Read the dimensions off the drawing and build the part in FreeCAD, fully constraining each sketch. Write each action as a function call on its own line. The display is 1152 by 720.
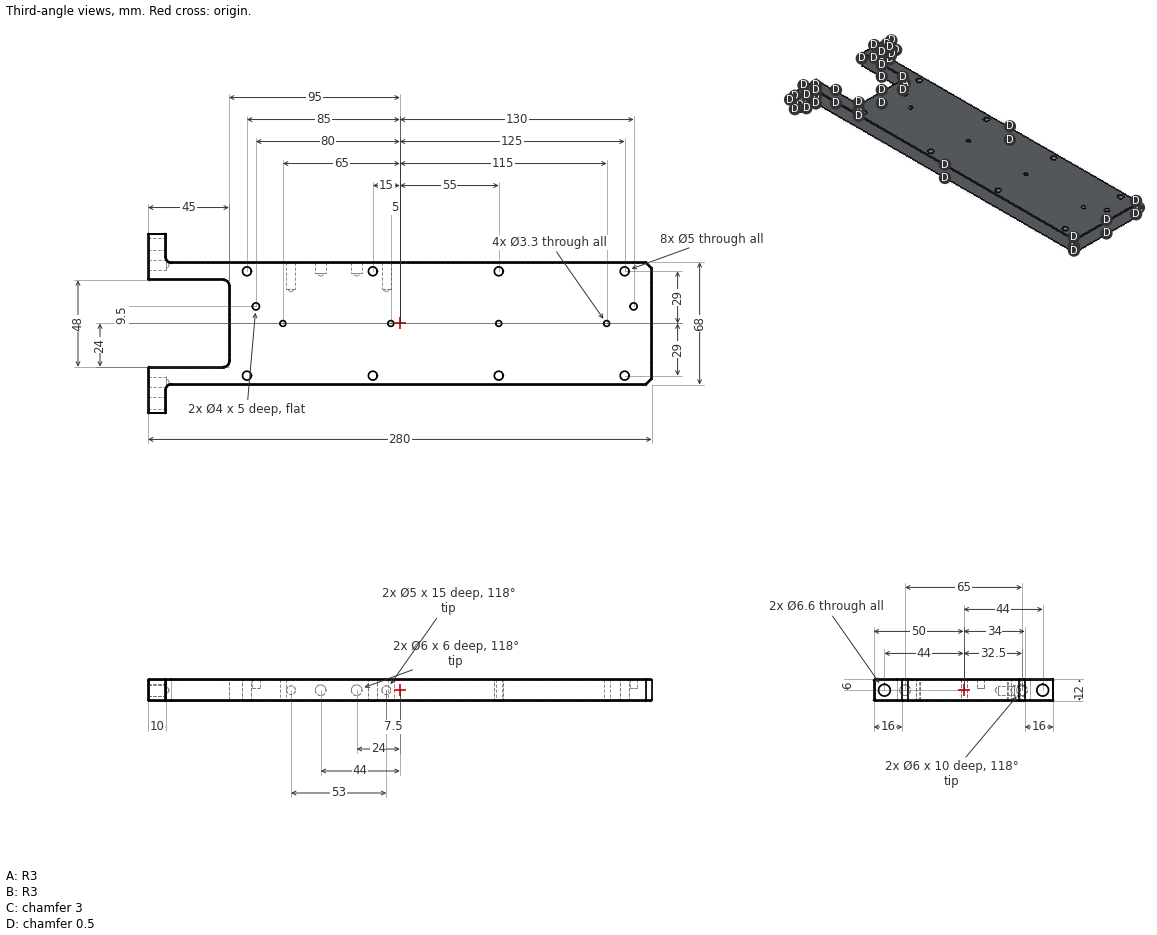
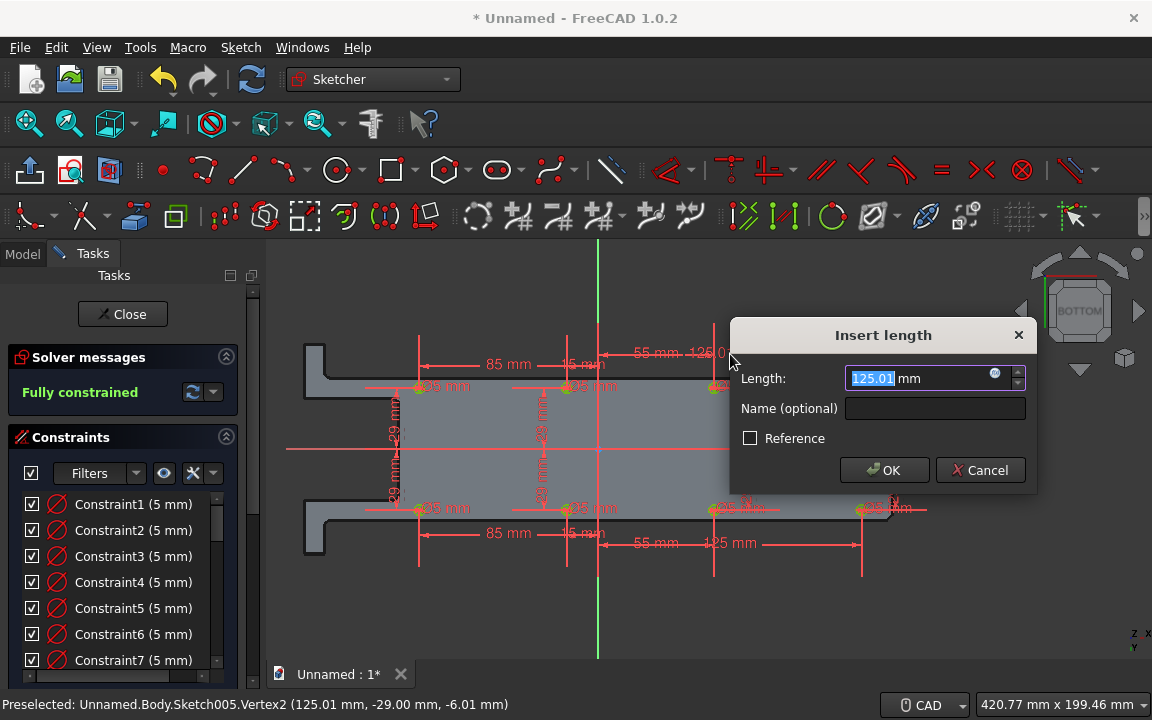
text(125)
key(Return)
key(Escape)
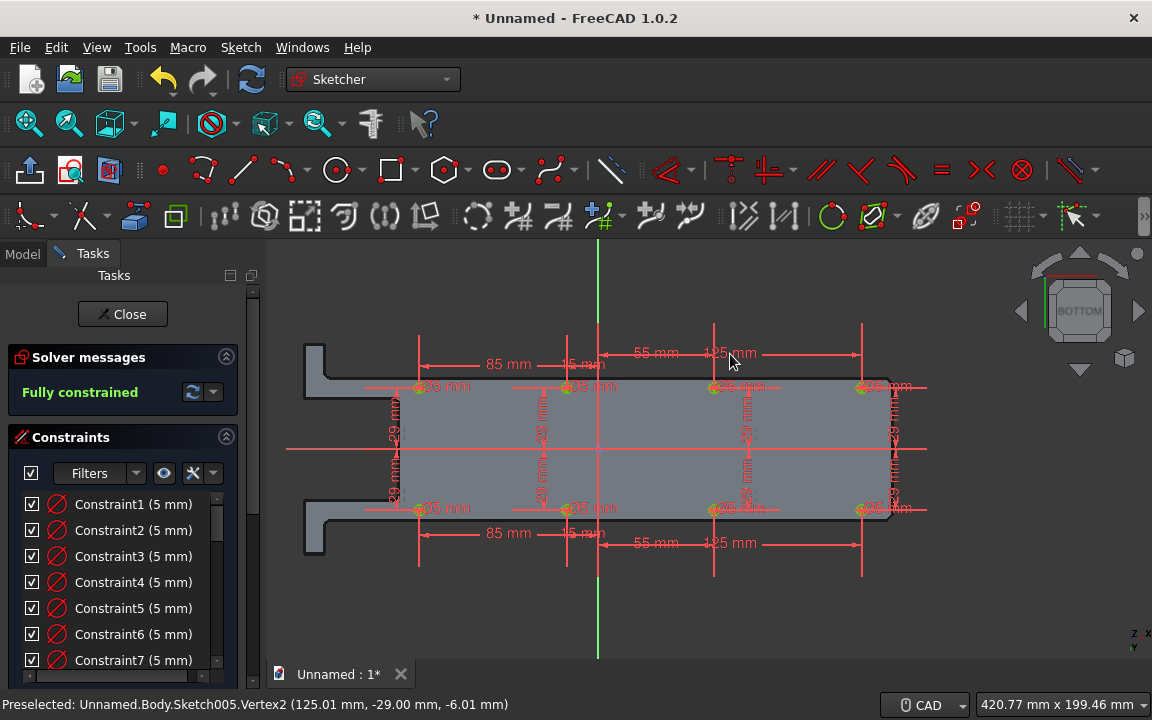
click(123, 314)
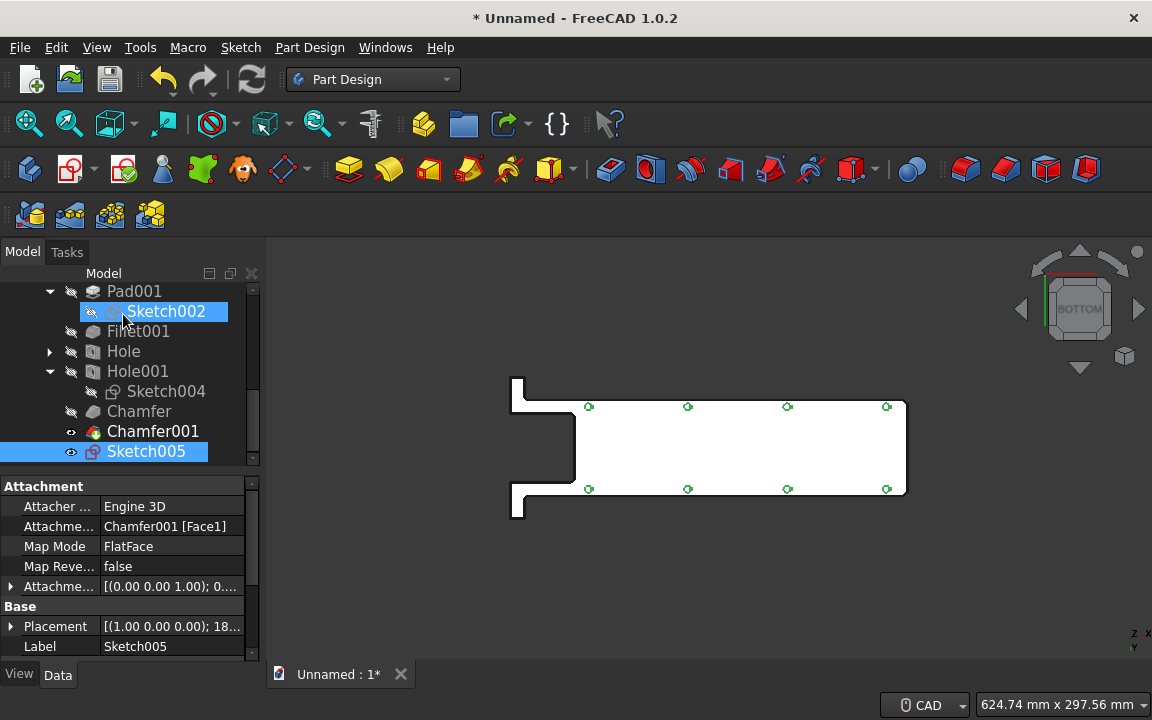
click(652, 170)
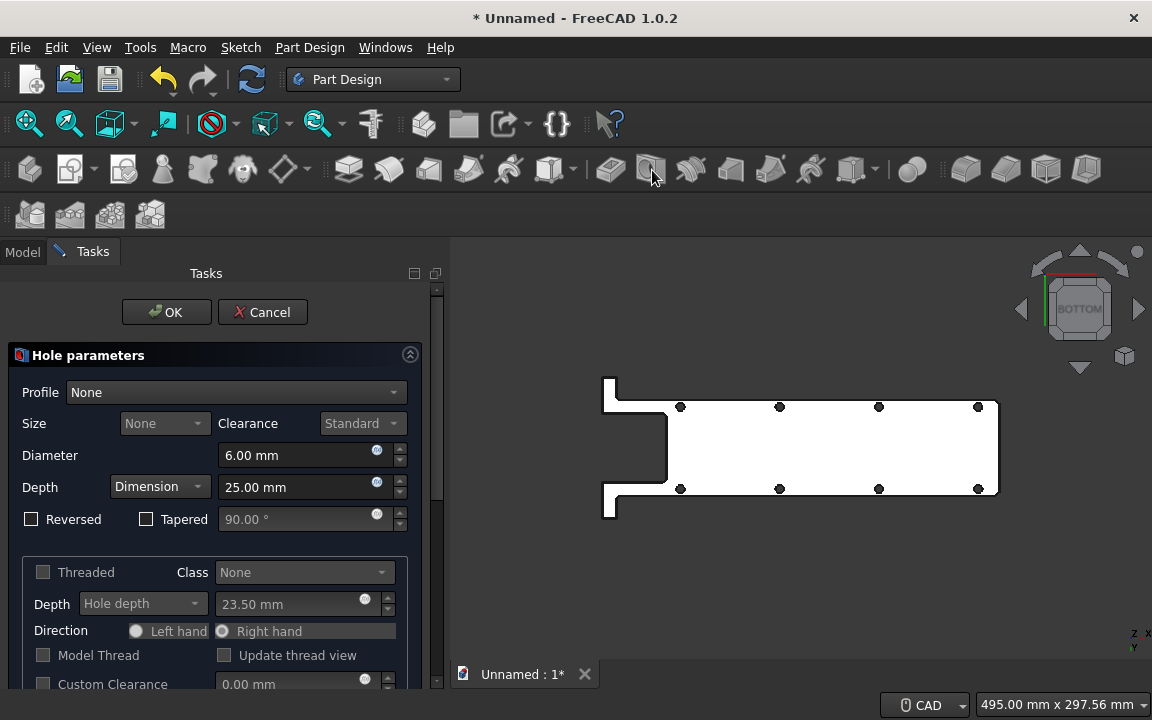
triple_click(305, 455)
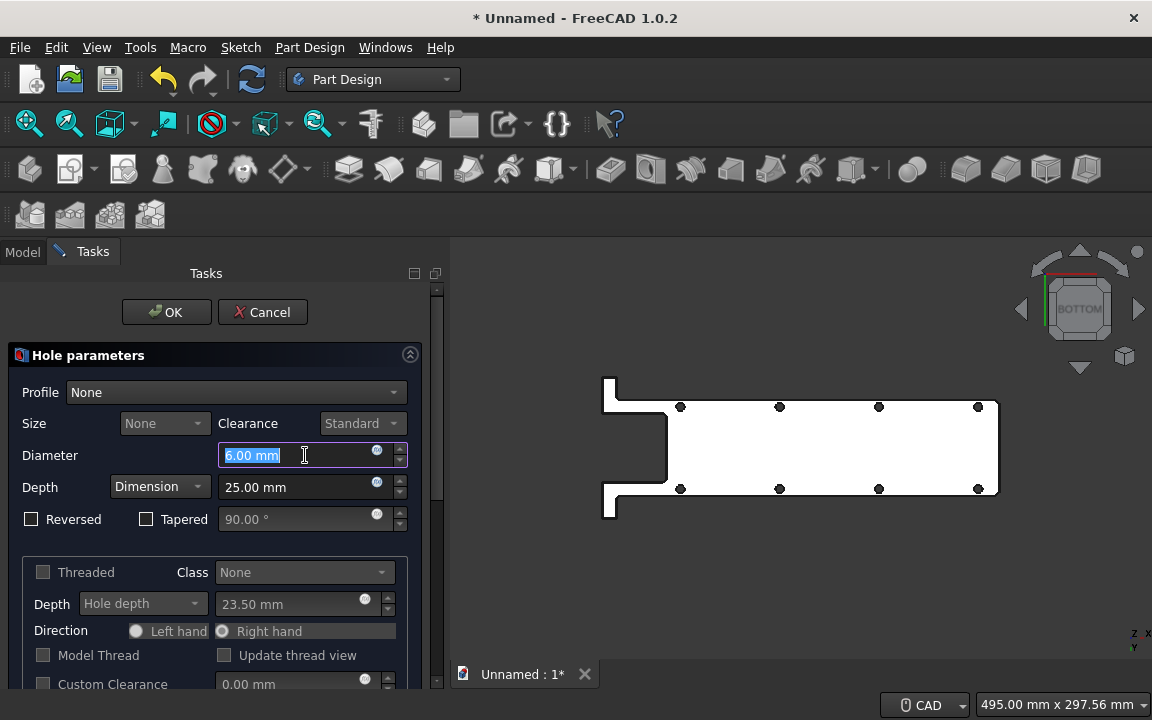
text(5)
key(Tab)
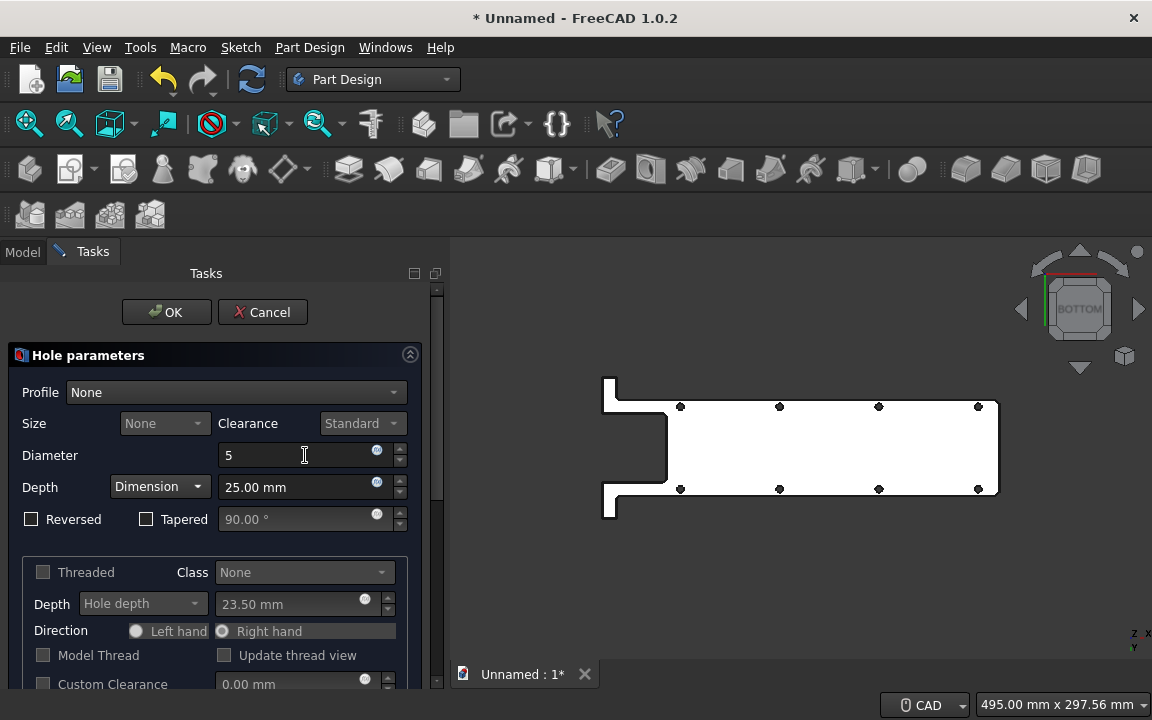
click(161, 486)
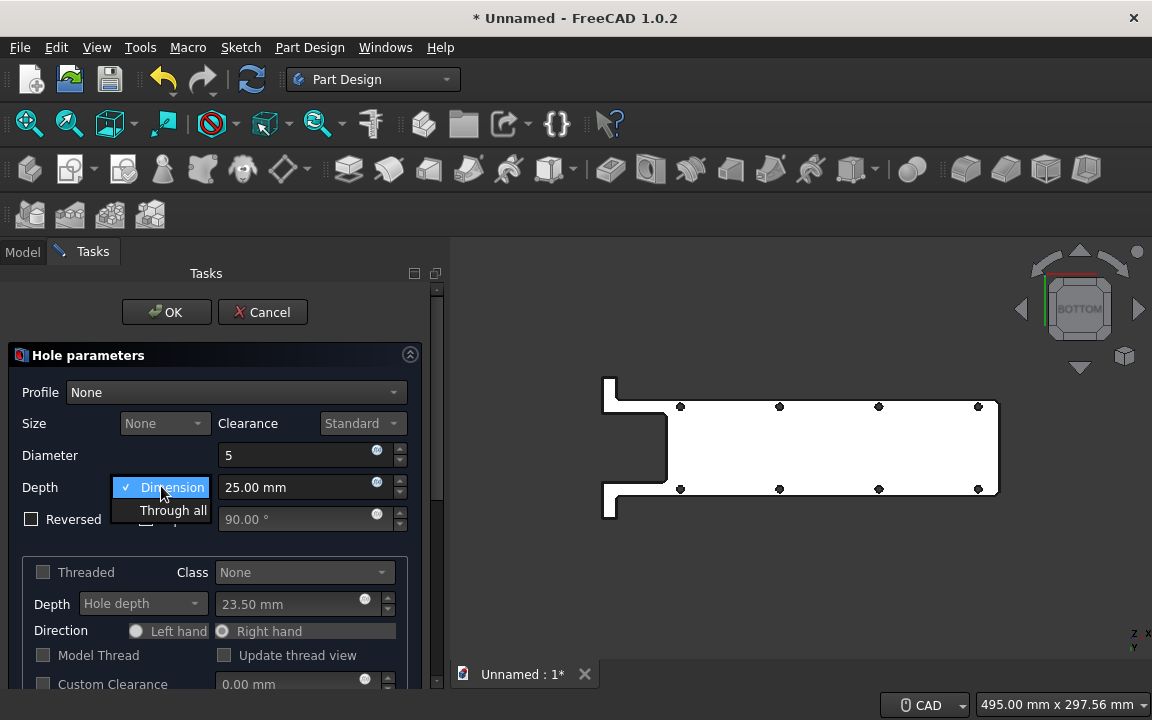
click(160, 510)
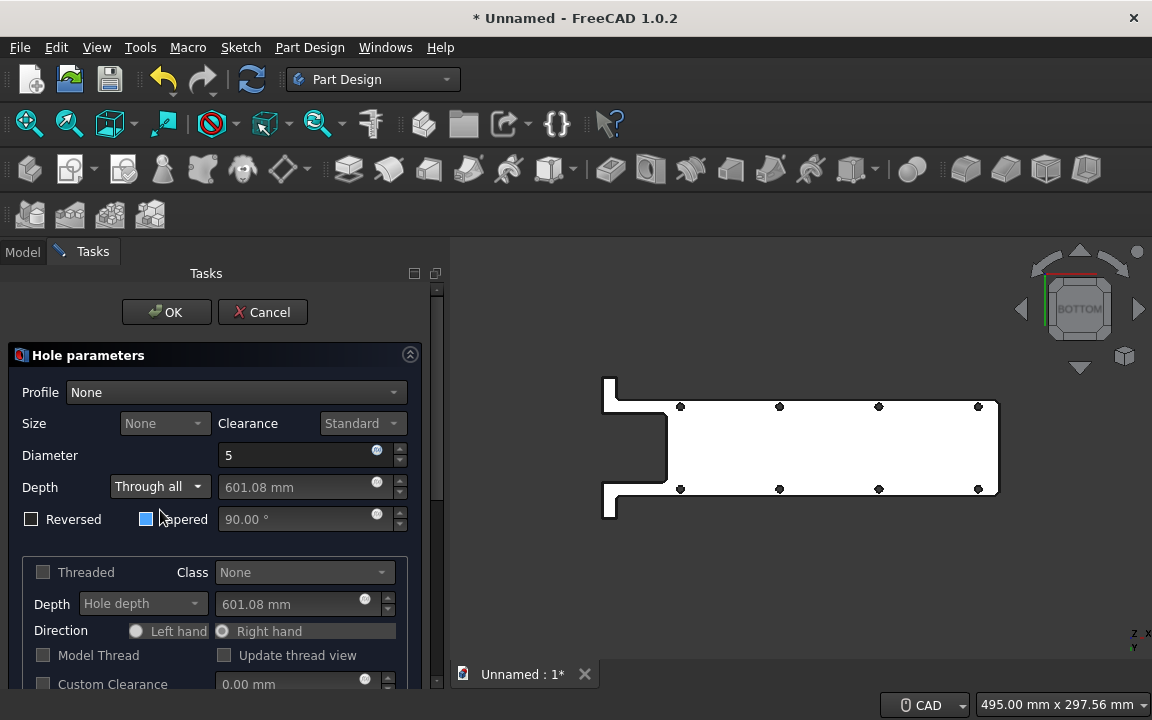
click(167, 312)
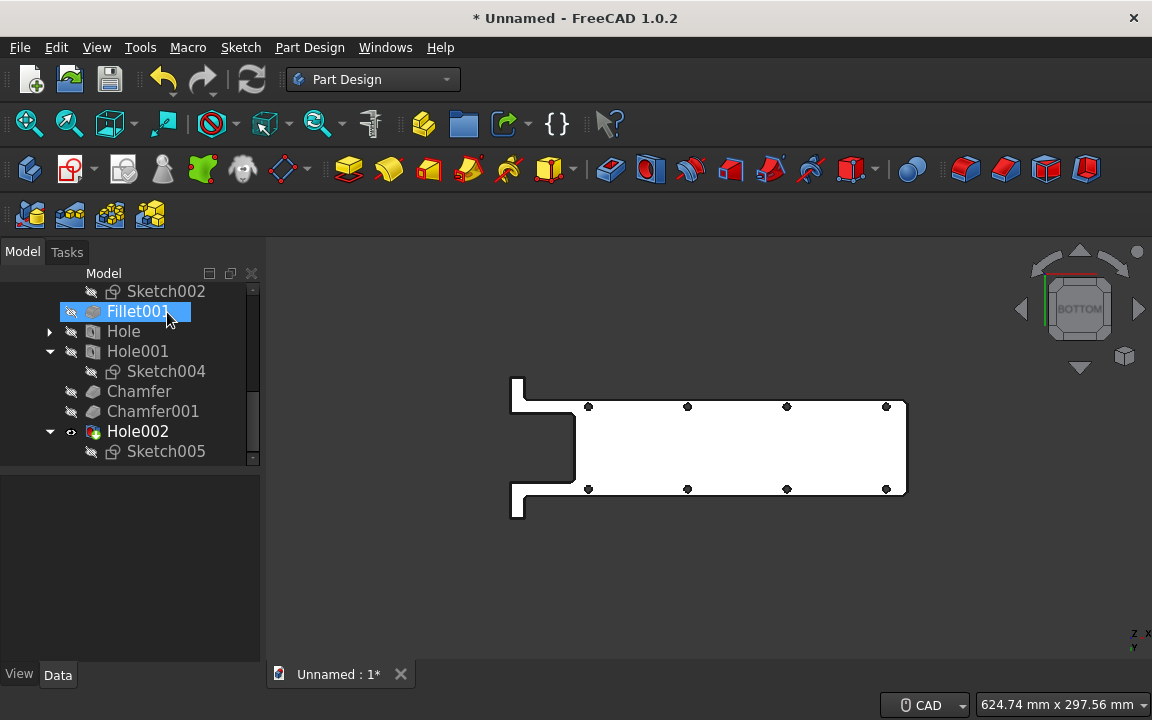
key(v)
key(f)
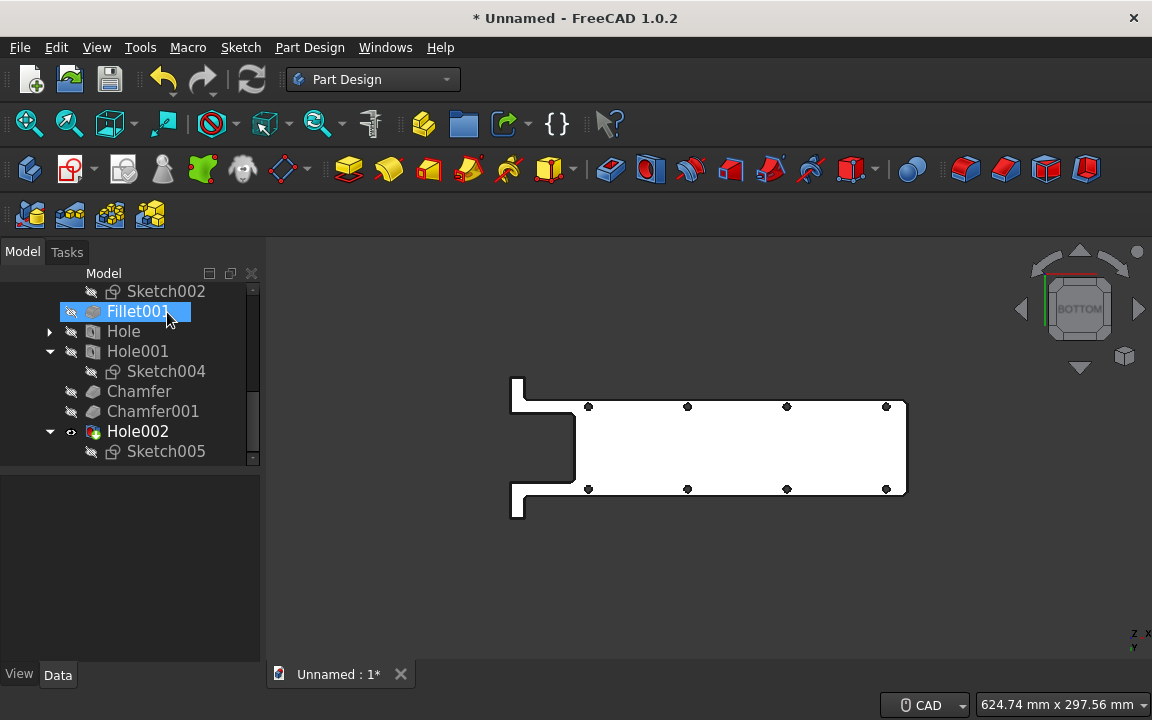
key(4)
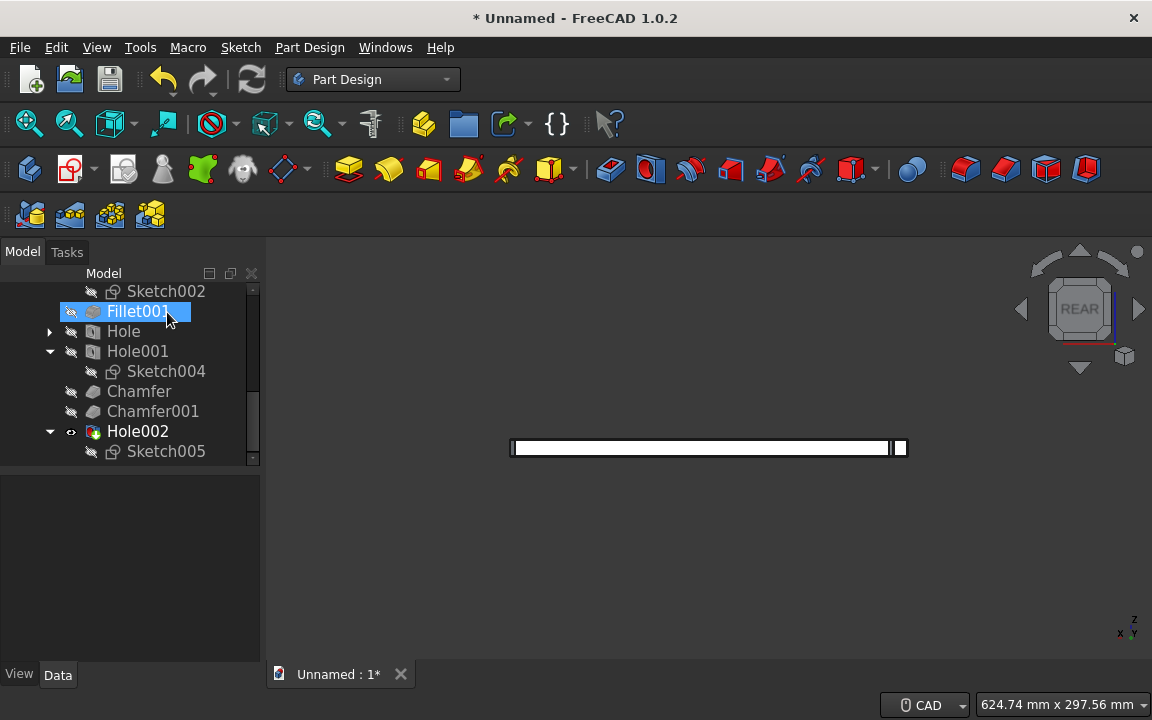
key(v)
key(f)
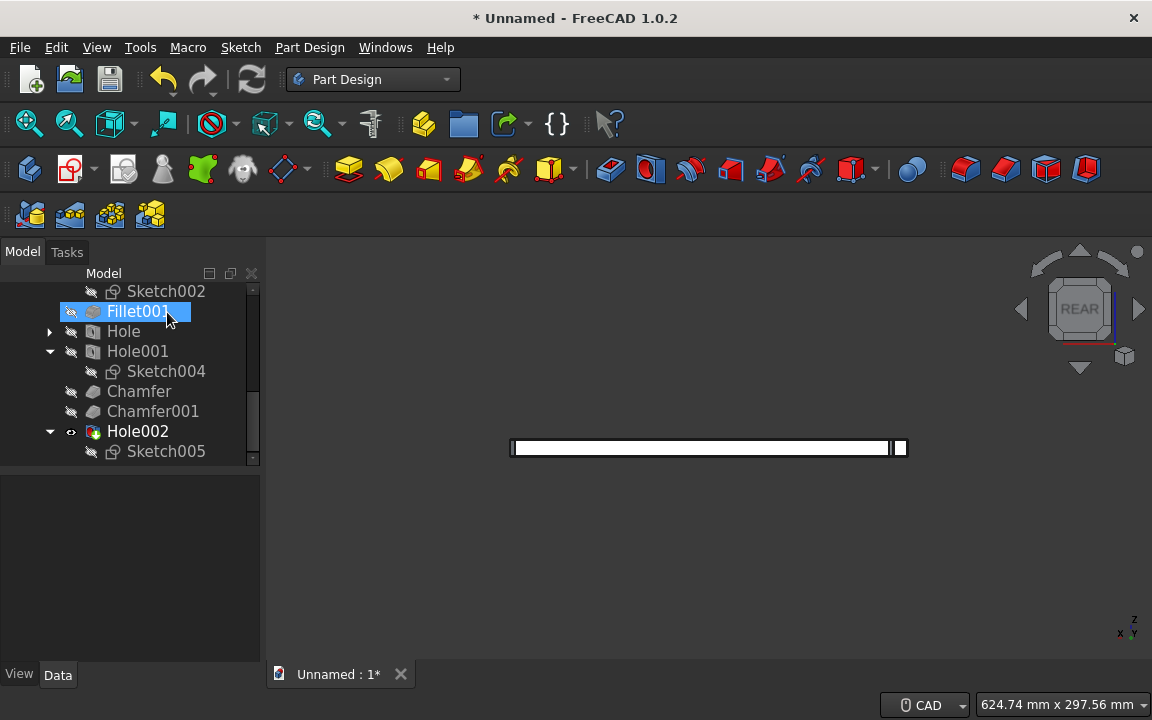
key(2)